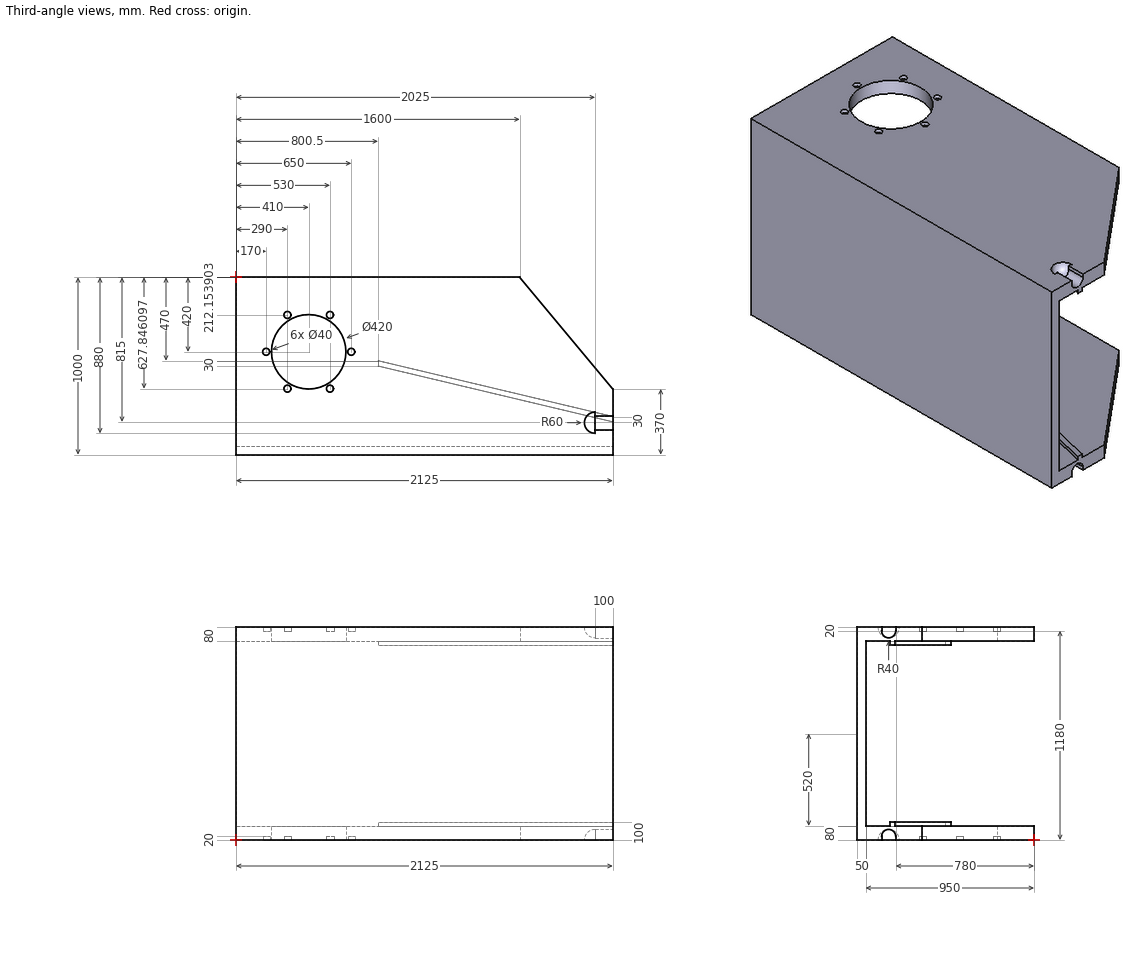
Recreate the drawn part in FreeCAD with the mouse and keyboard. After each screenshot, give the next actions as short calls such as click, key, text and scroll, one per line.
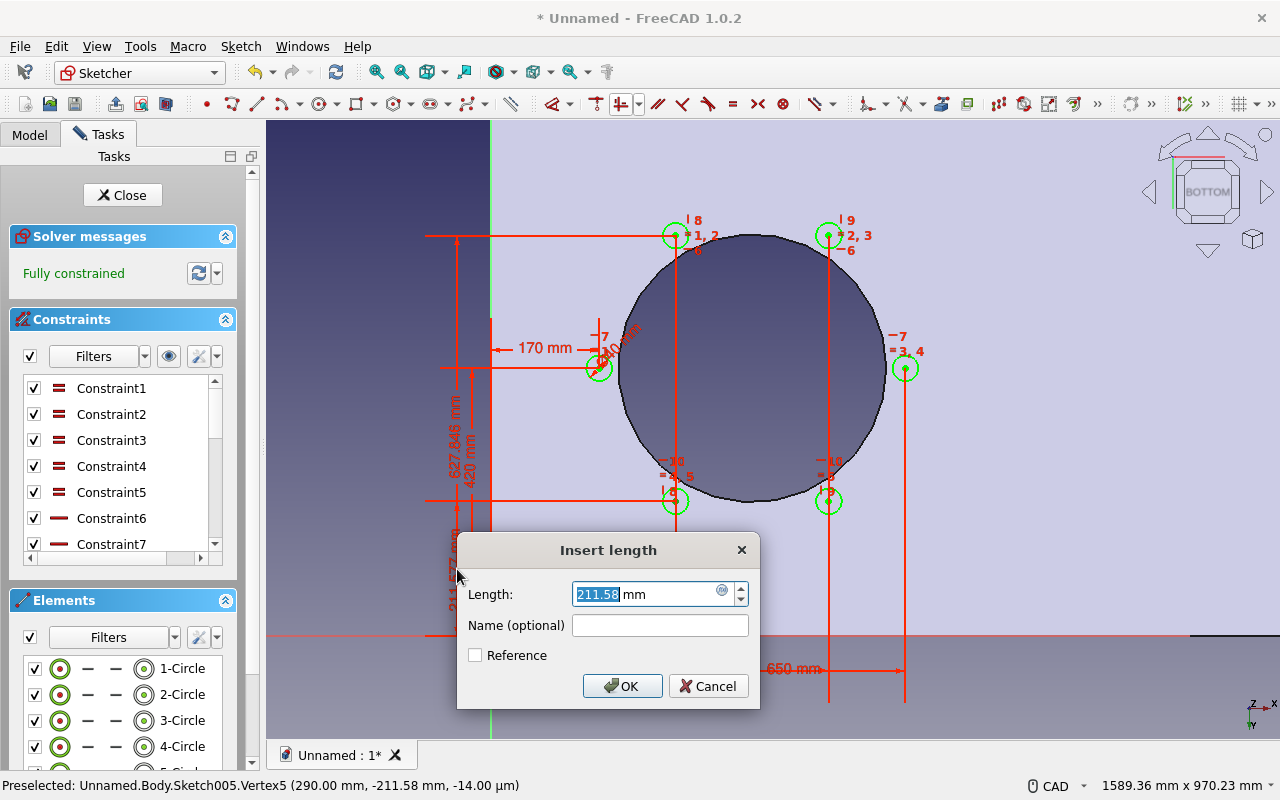
text(212.153903)
key(Return)
key(Escape)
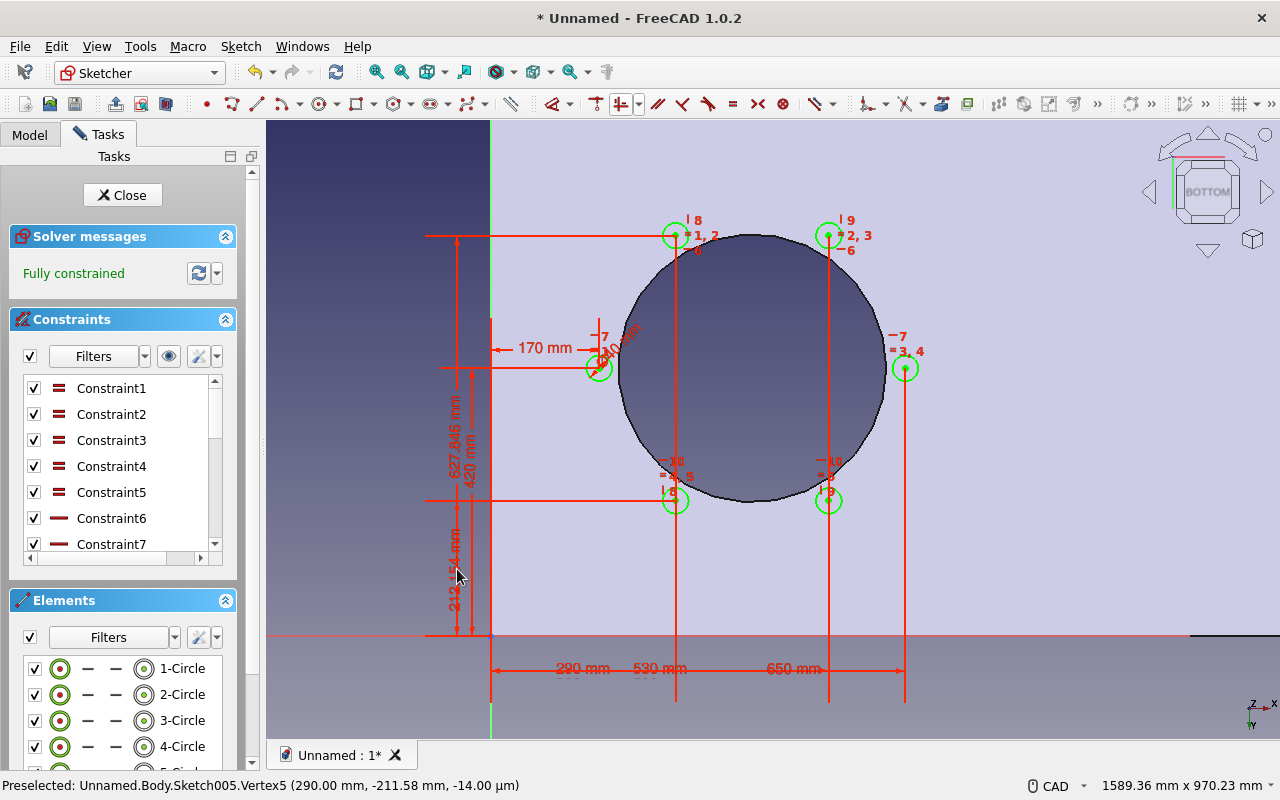
click(123, 195)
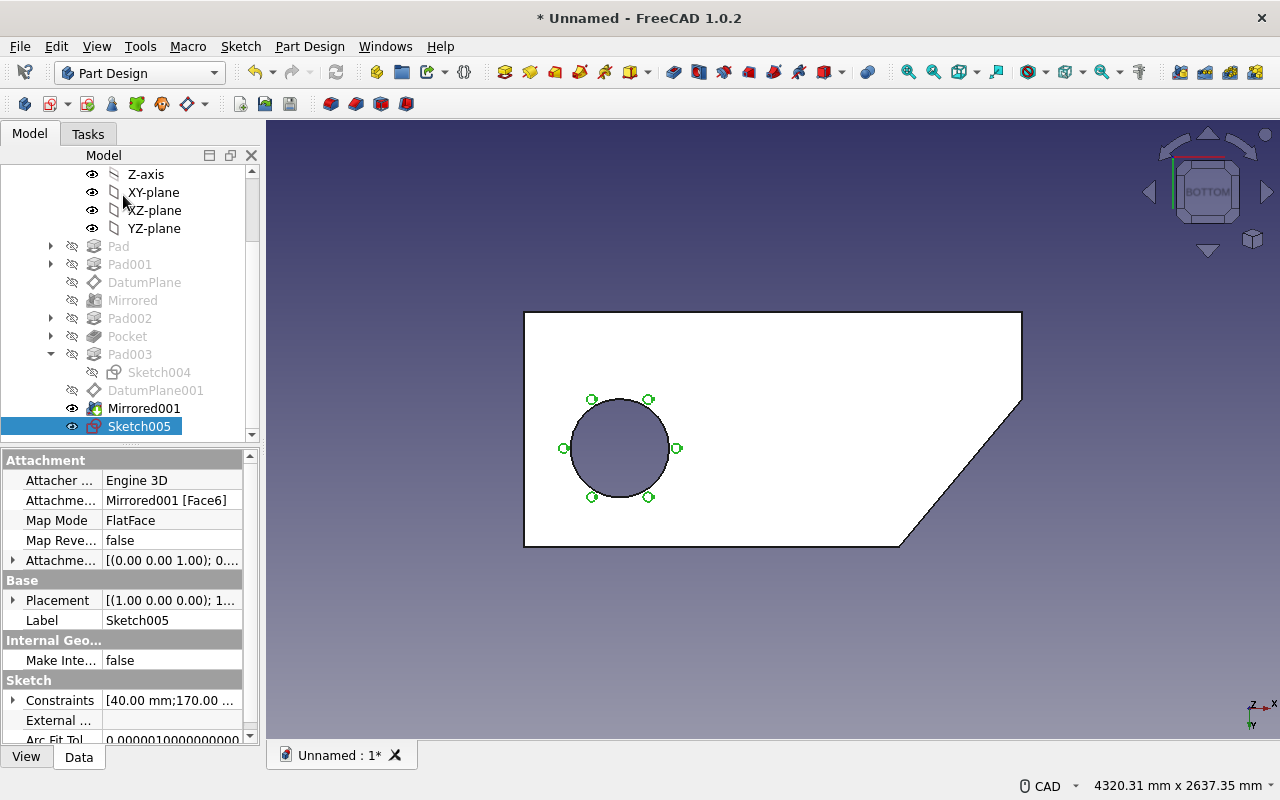
click(674, 72)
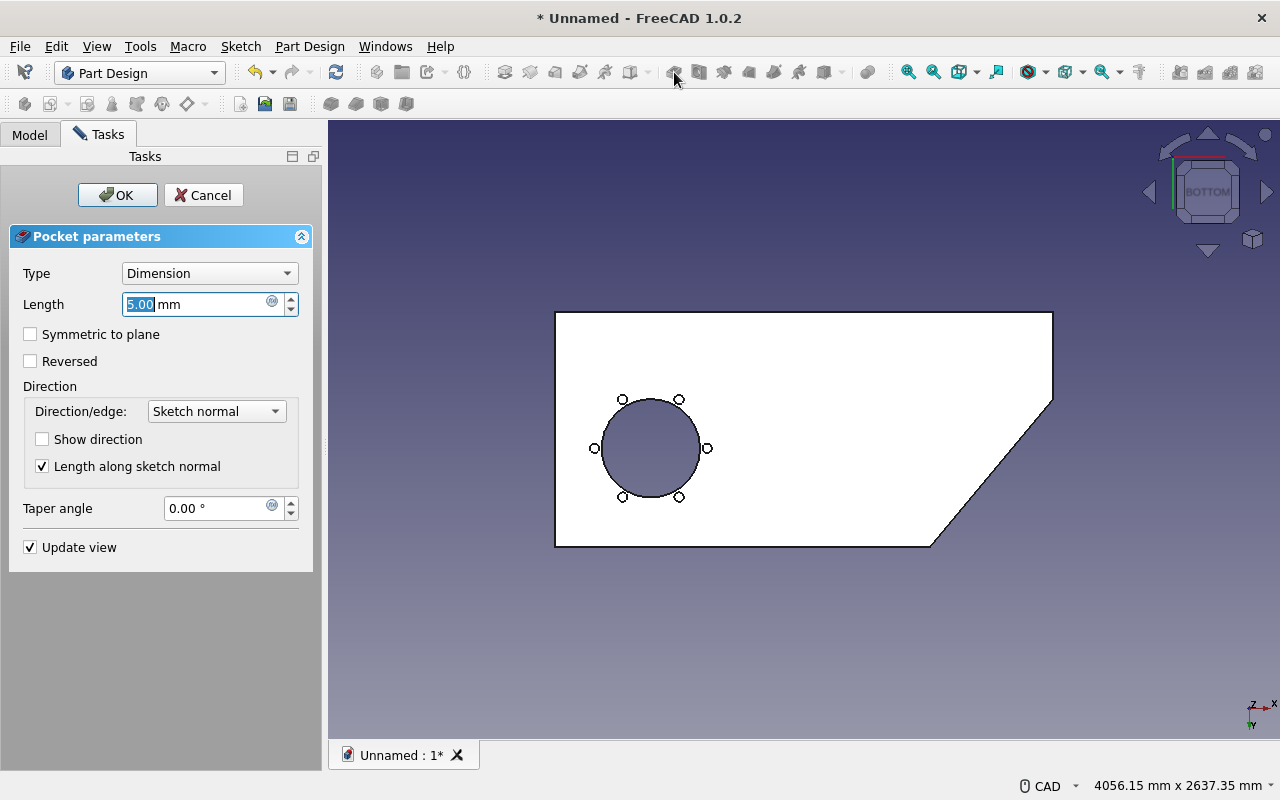
text(20)
key(Tab)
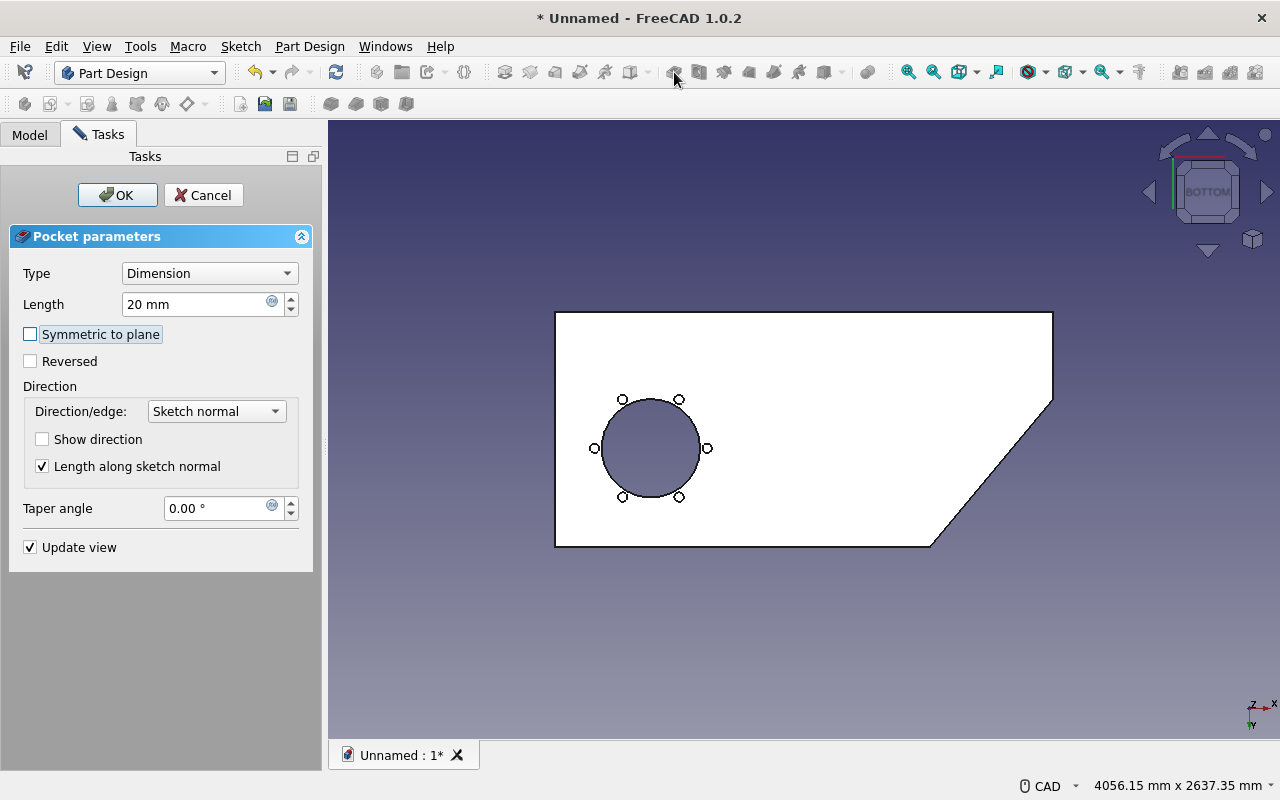
click(118, 195)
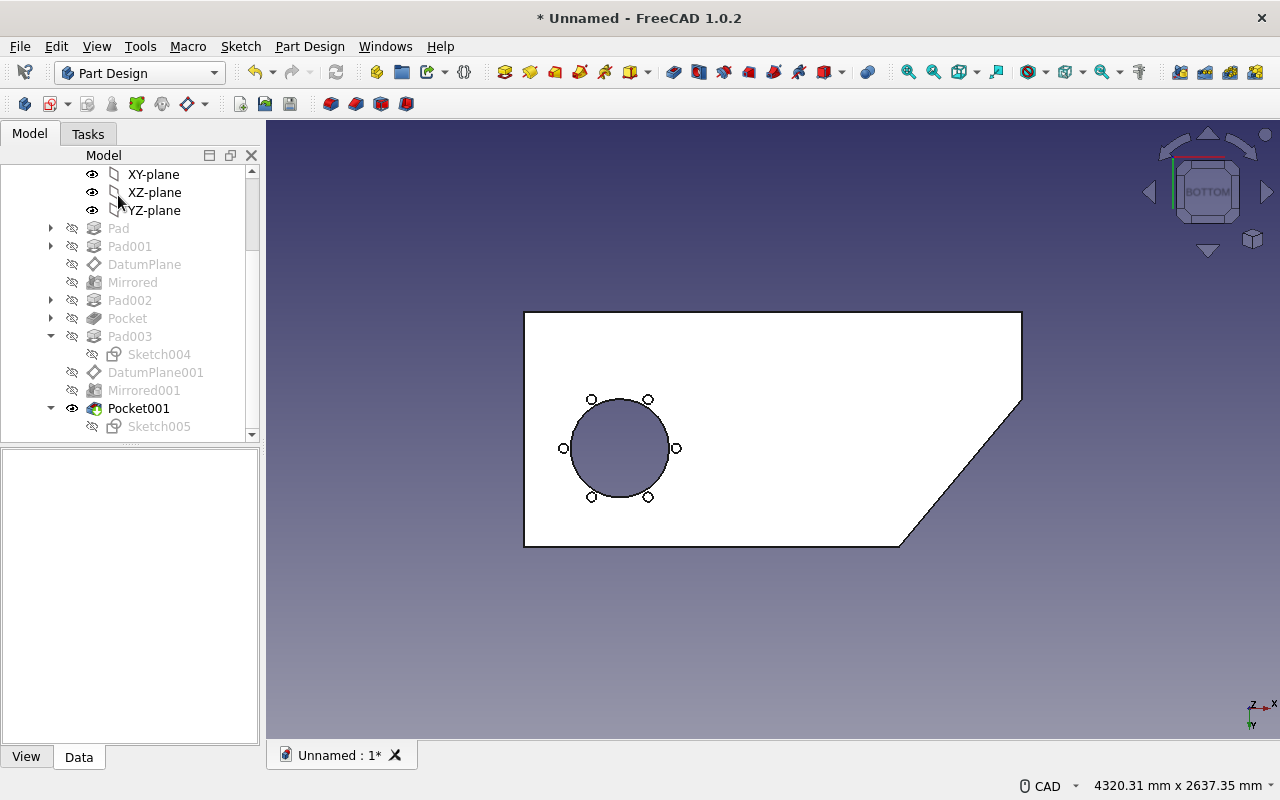
scroll(161, 296, down, 3)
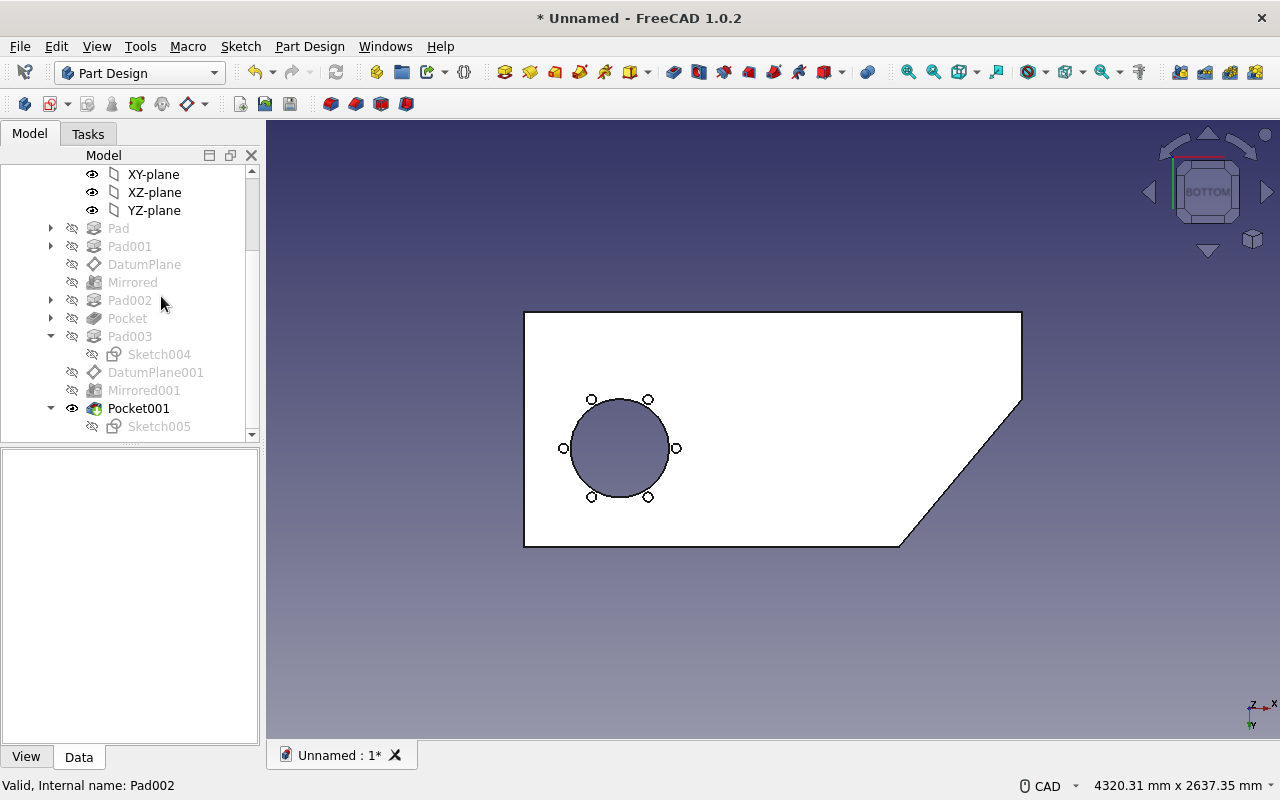
scroll(161, 296, up, 15)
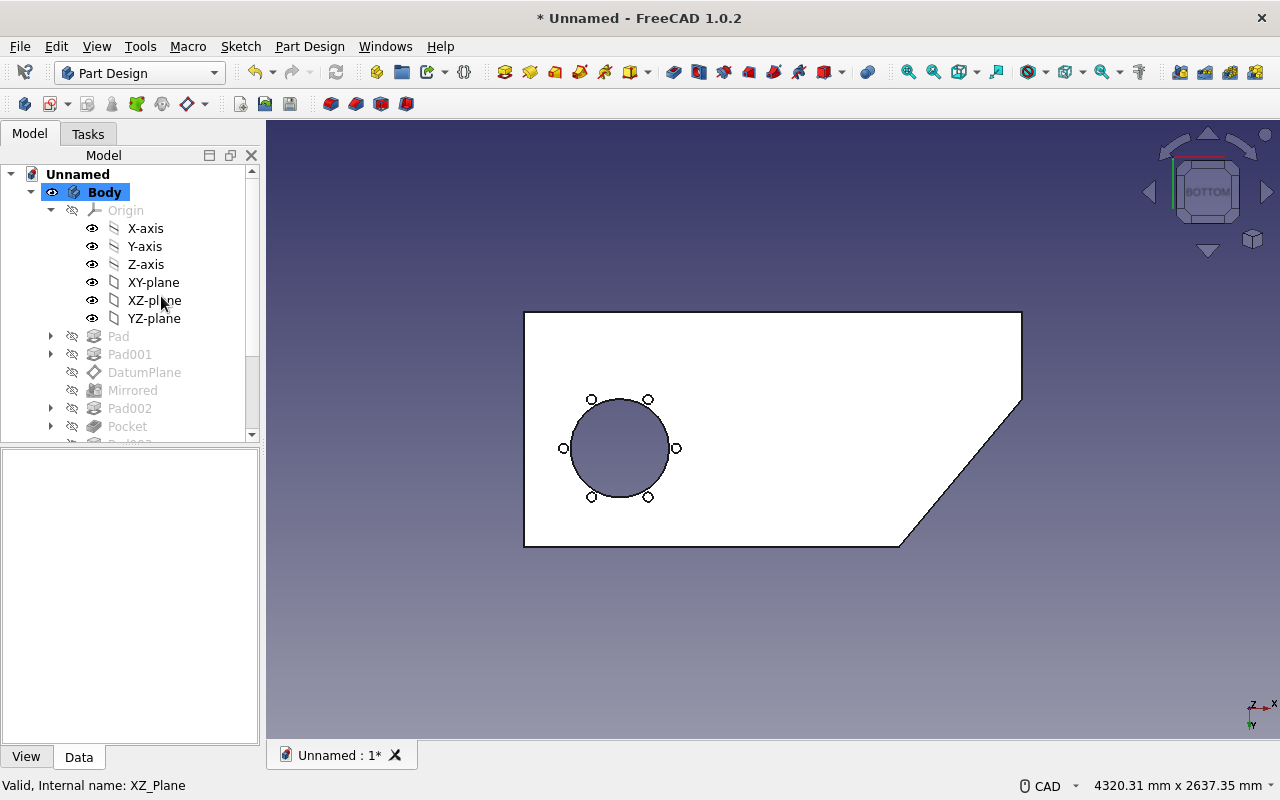
click(137, 282)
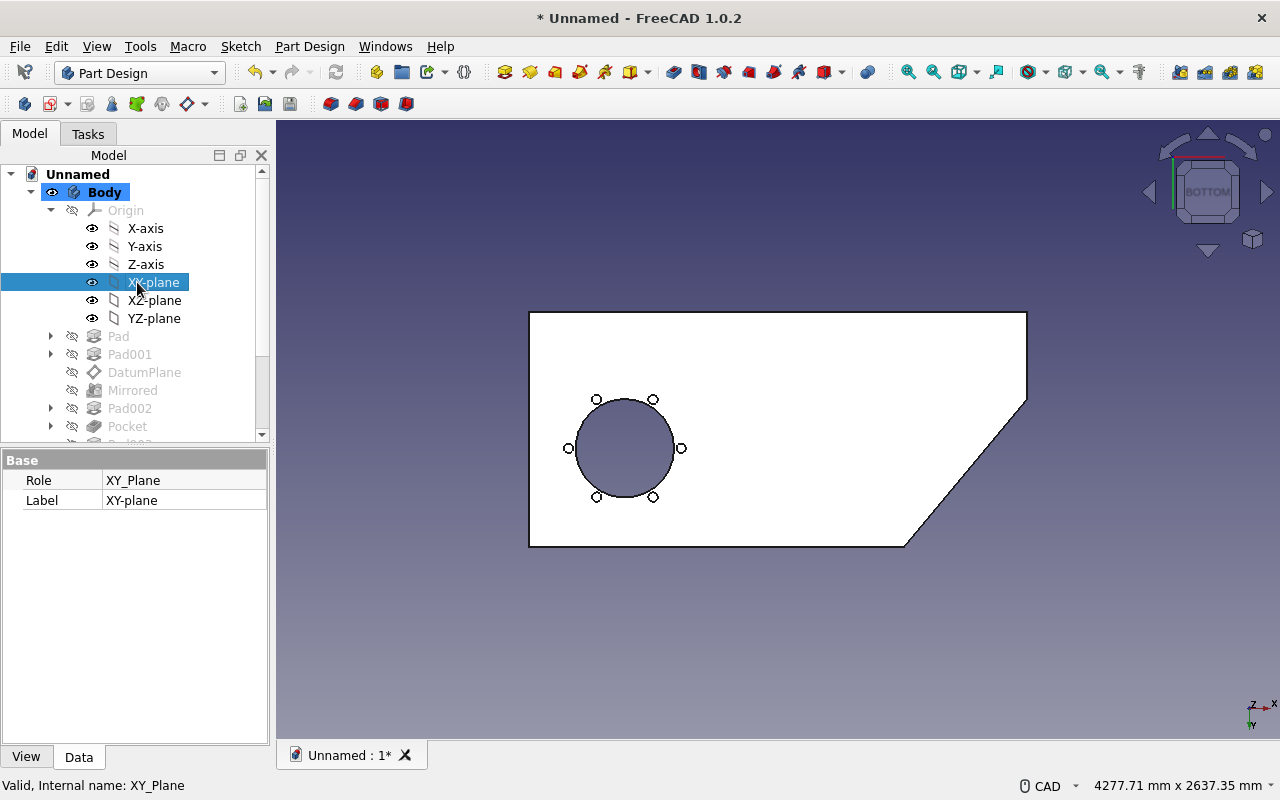
click(186, 104)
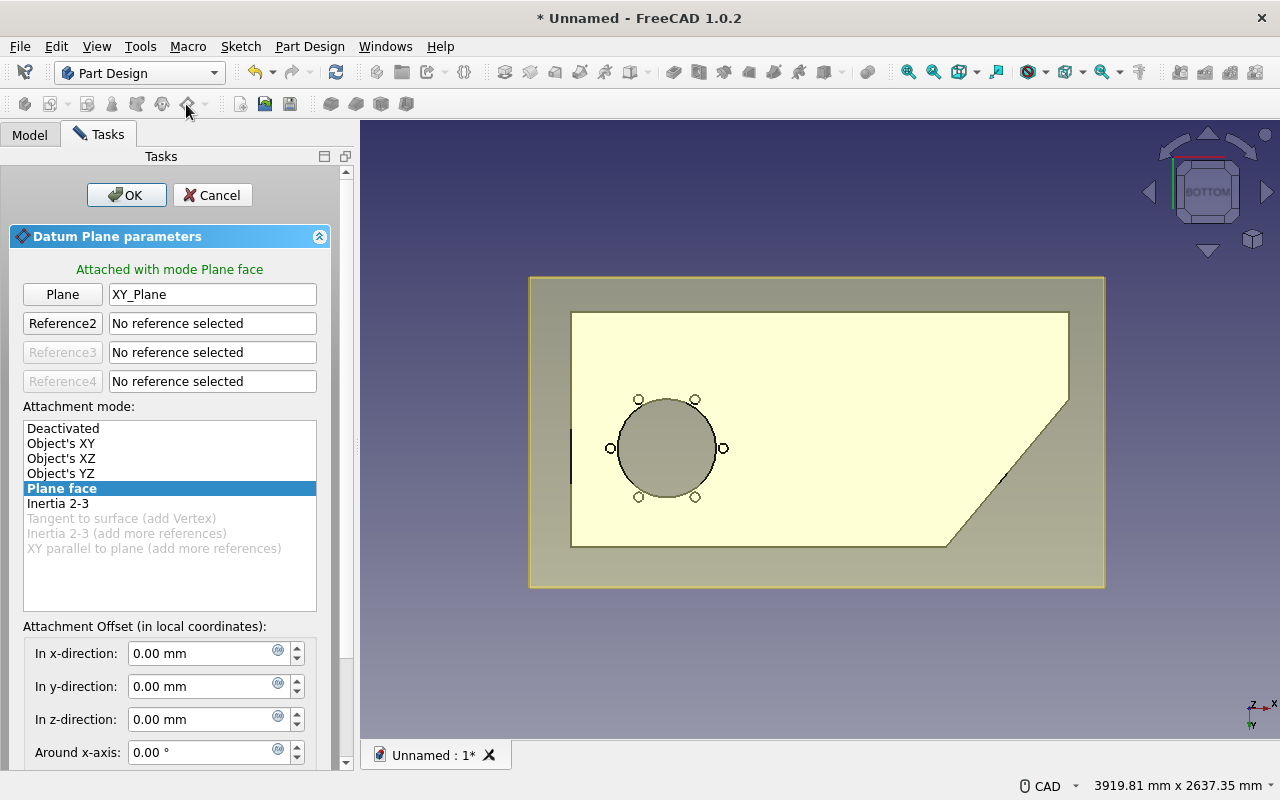
triple_click(210, 720)